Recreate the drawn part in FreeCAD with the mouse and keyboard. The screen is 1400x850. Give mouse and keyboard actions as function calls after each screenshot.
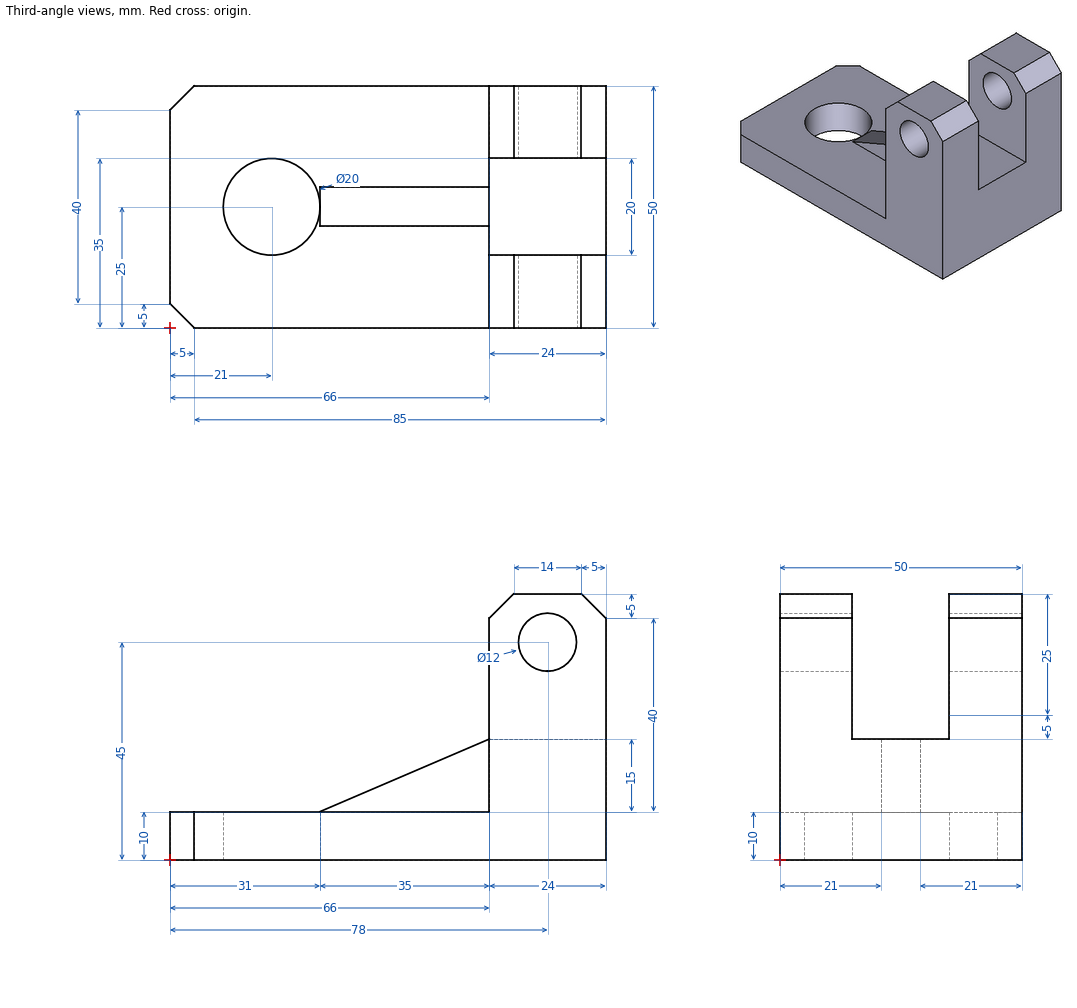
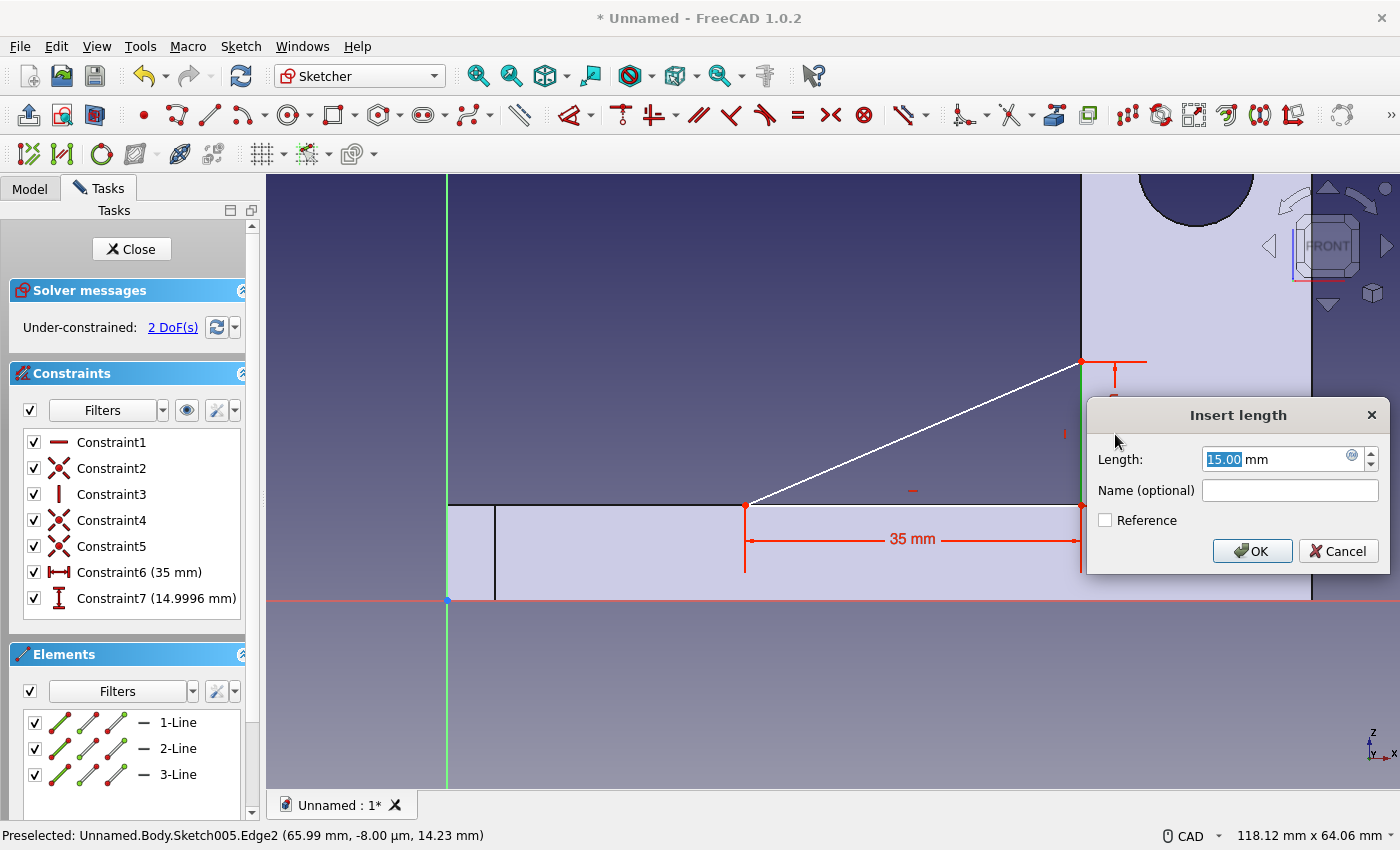
text(15)
key(Return)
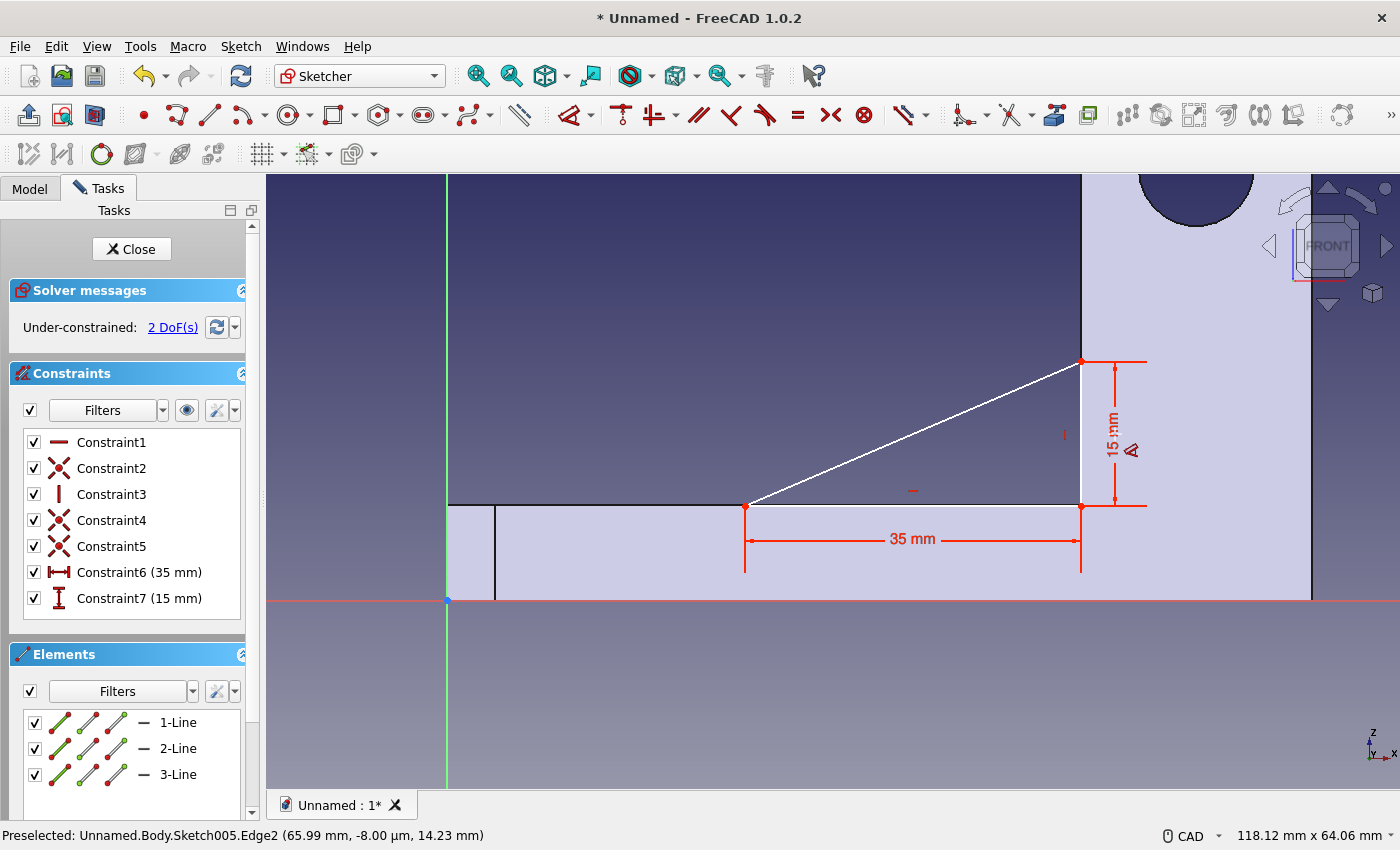
click(745, 506)
click(596, 635)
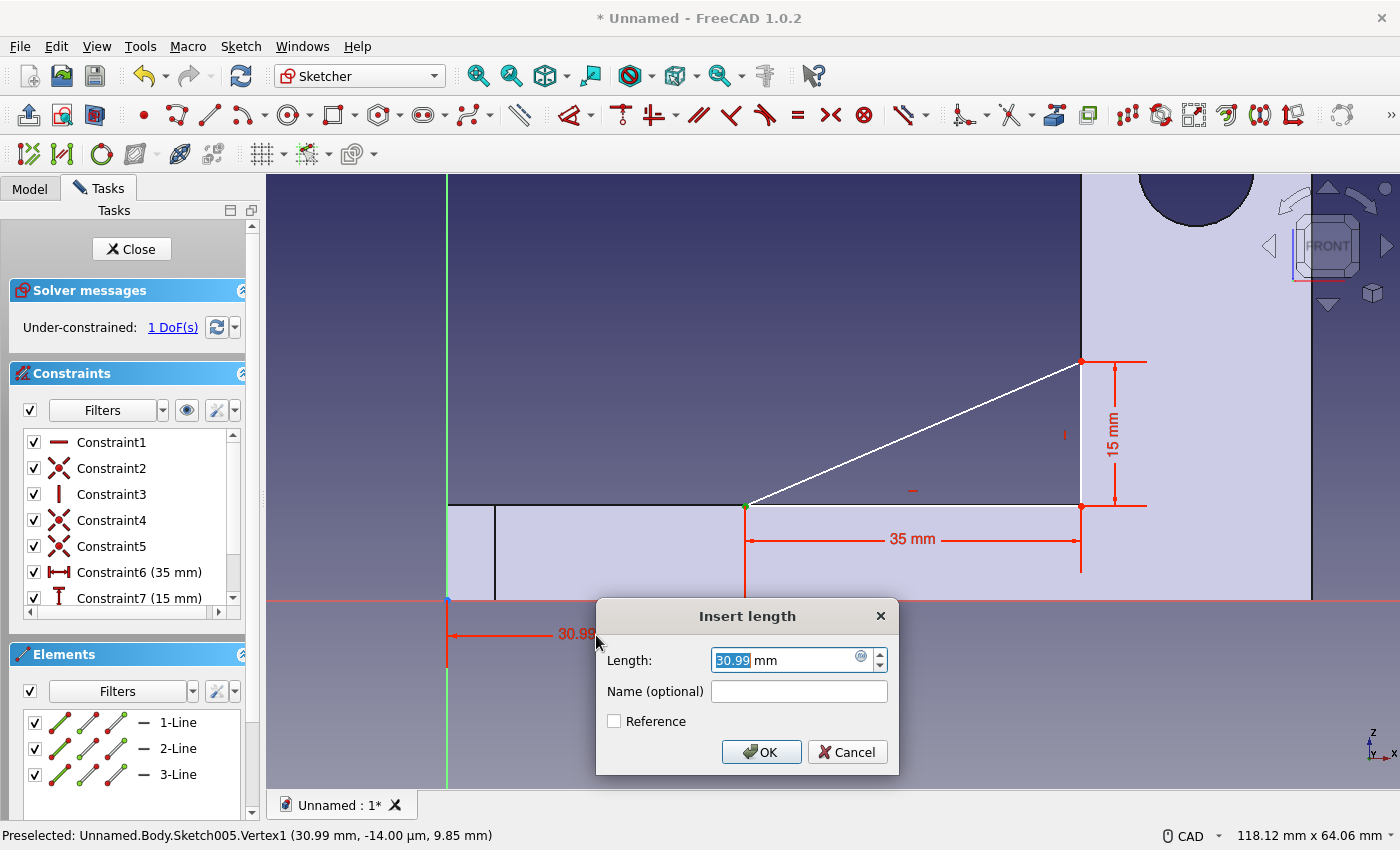
text(31)
key(Return)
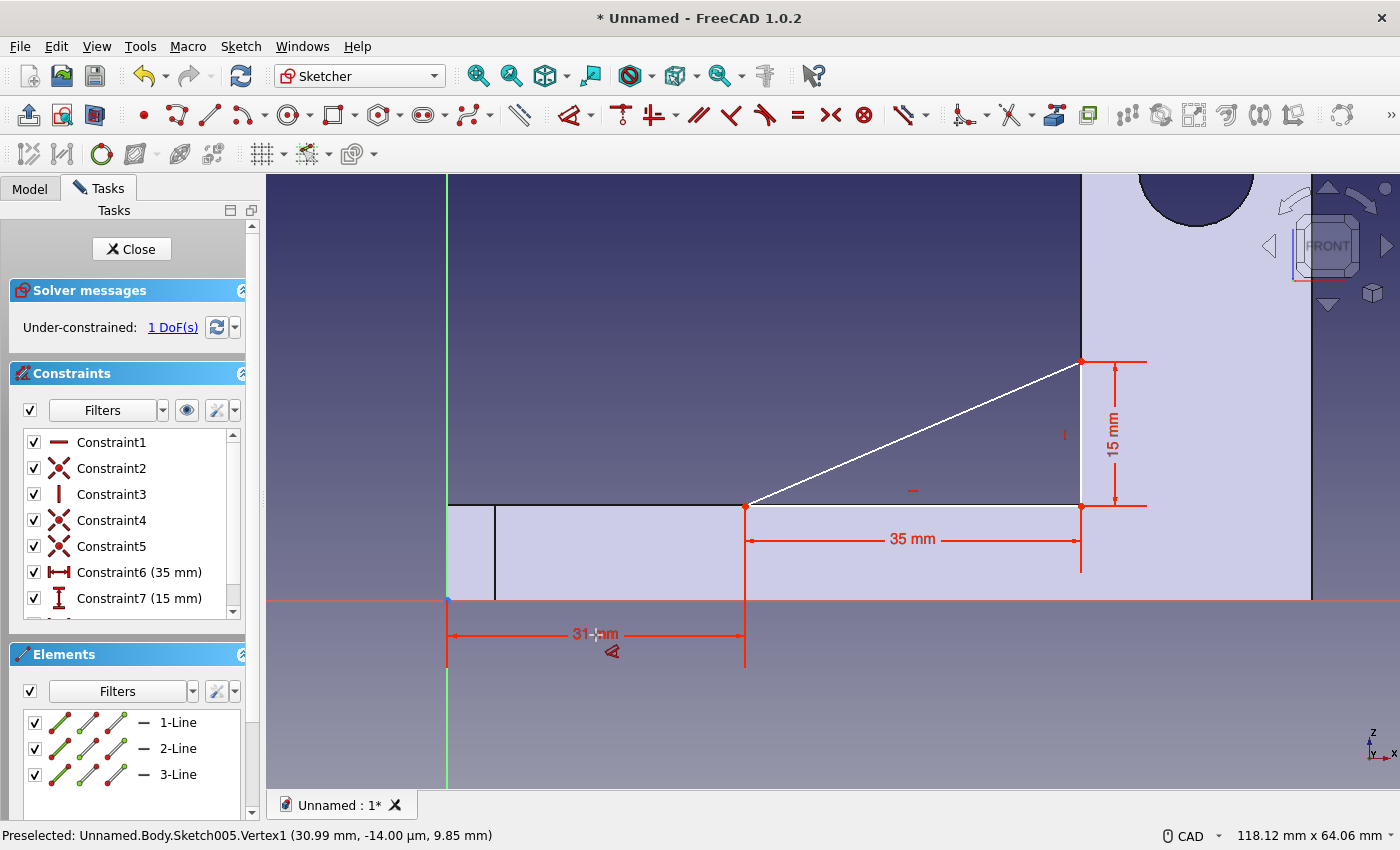
click(745, 506)
click(413, 553)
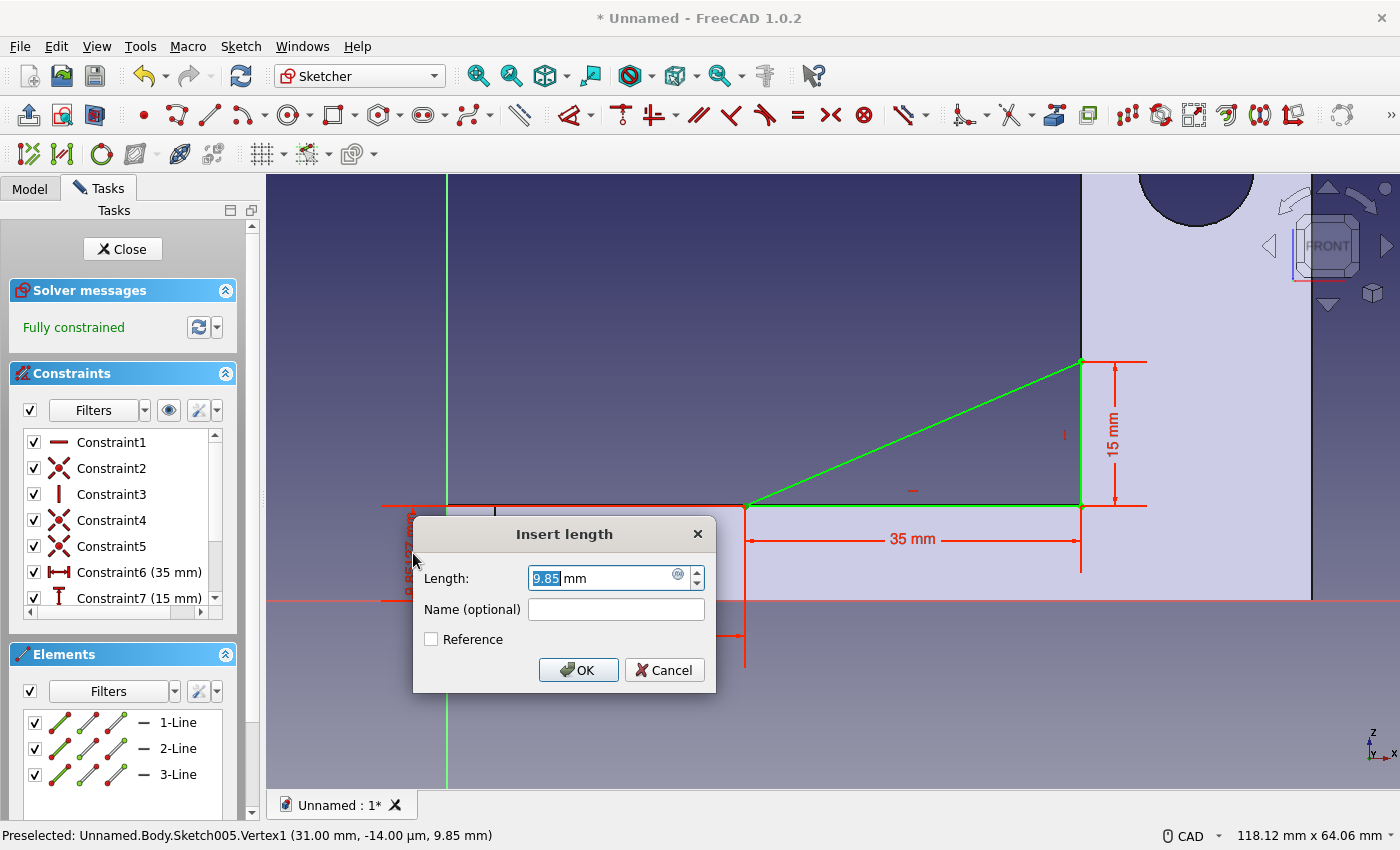
text(10)
key(Return)
key(Escape)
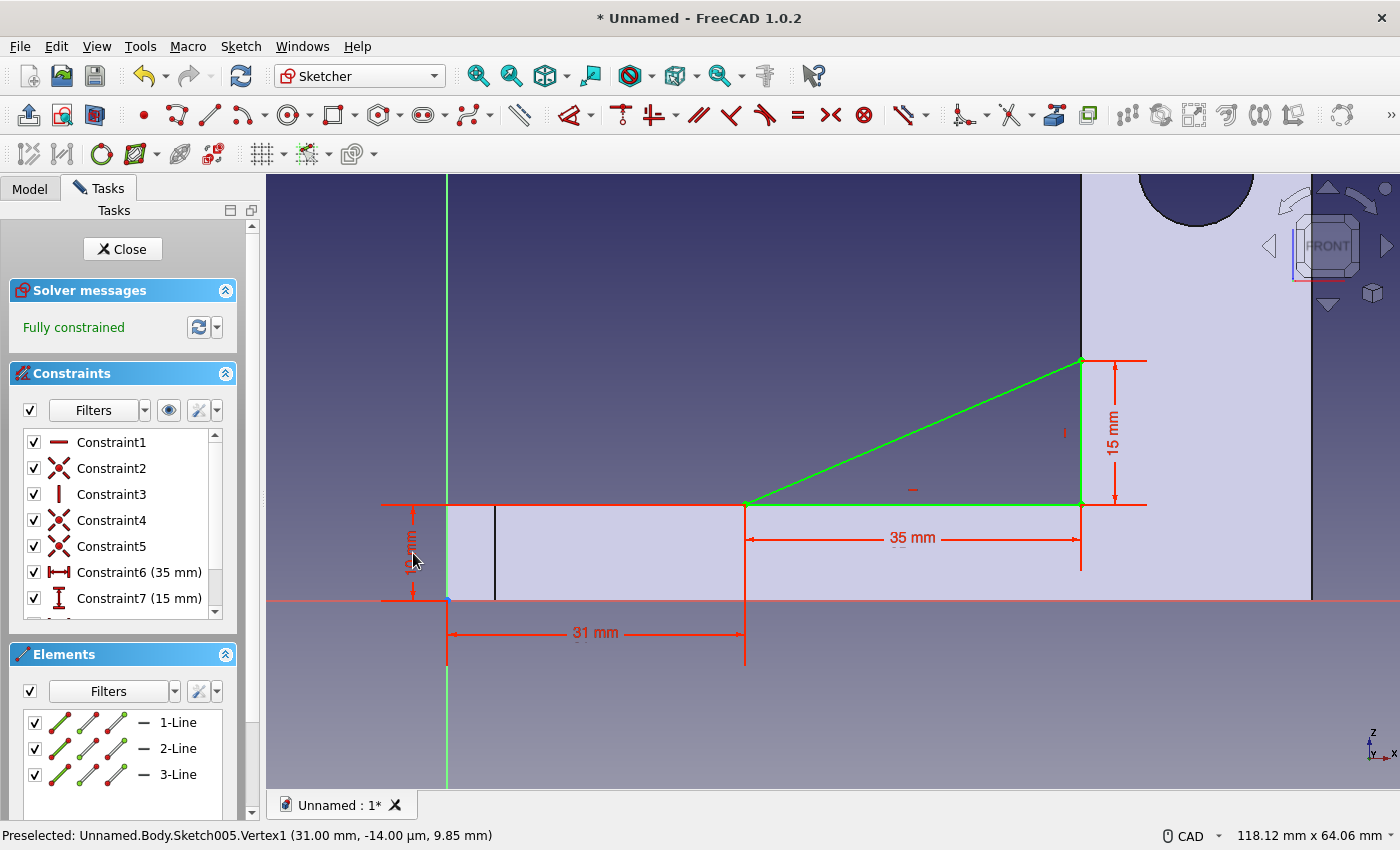
click(123, 249)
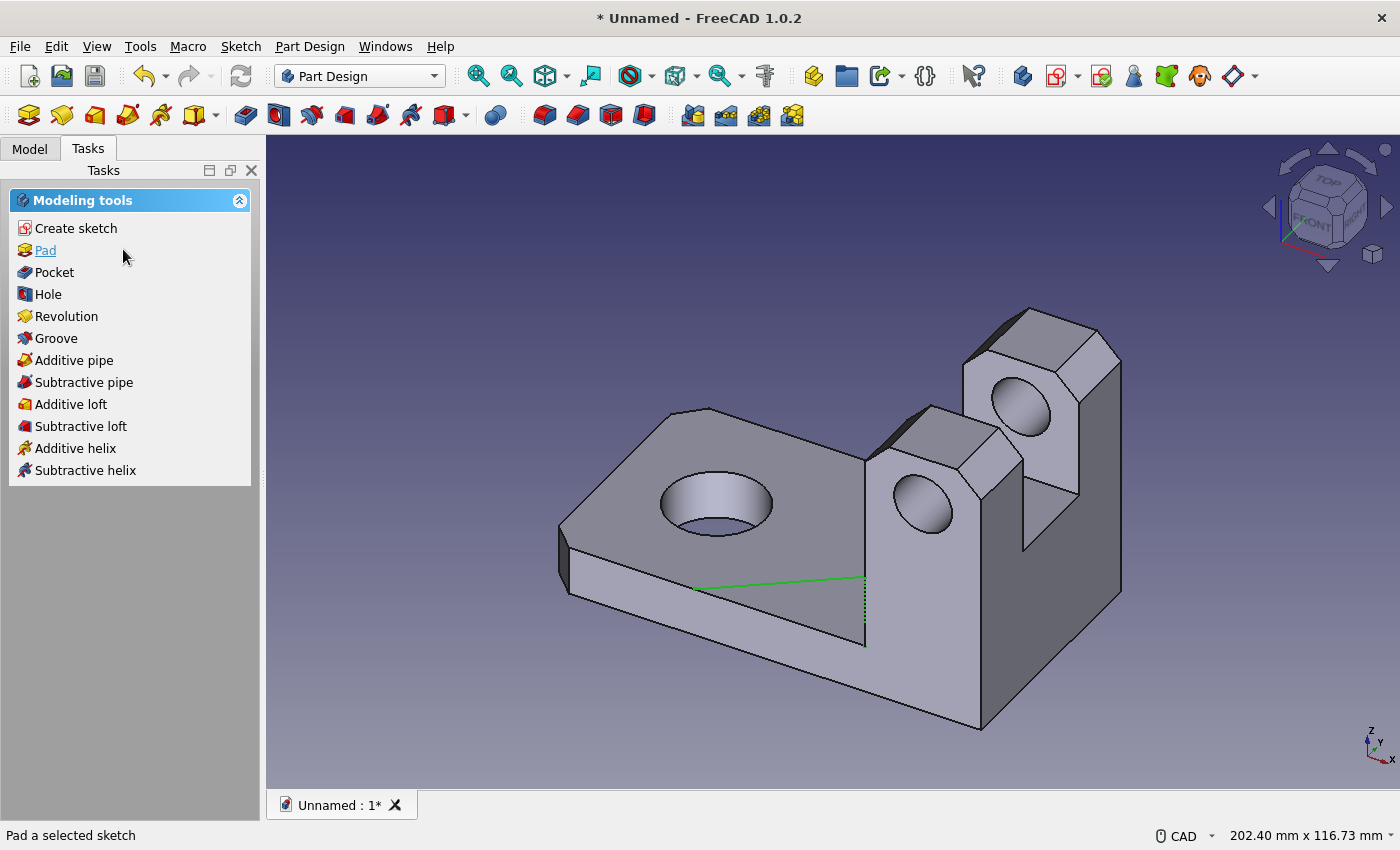
click(29, 116)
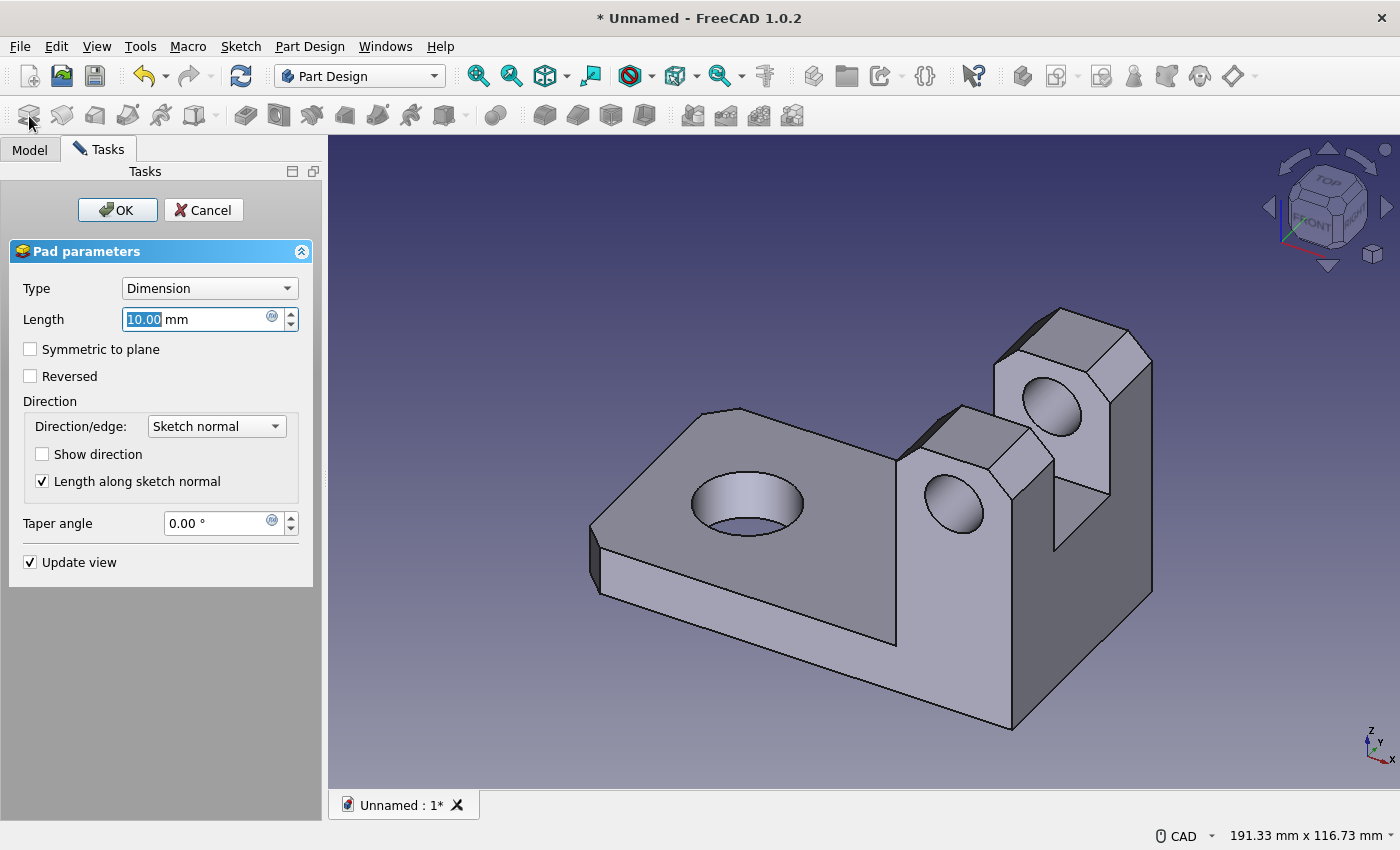
text(50)
key(Tab)